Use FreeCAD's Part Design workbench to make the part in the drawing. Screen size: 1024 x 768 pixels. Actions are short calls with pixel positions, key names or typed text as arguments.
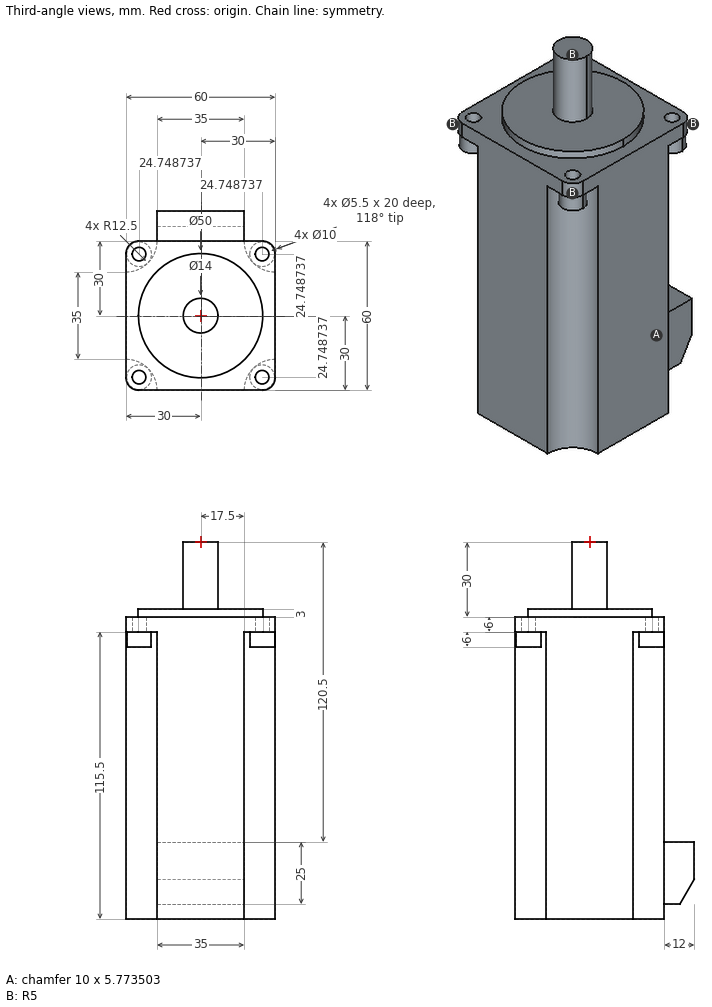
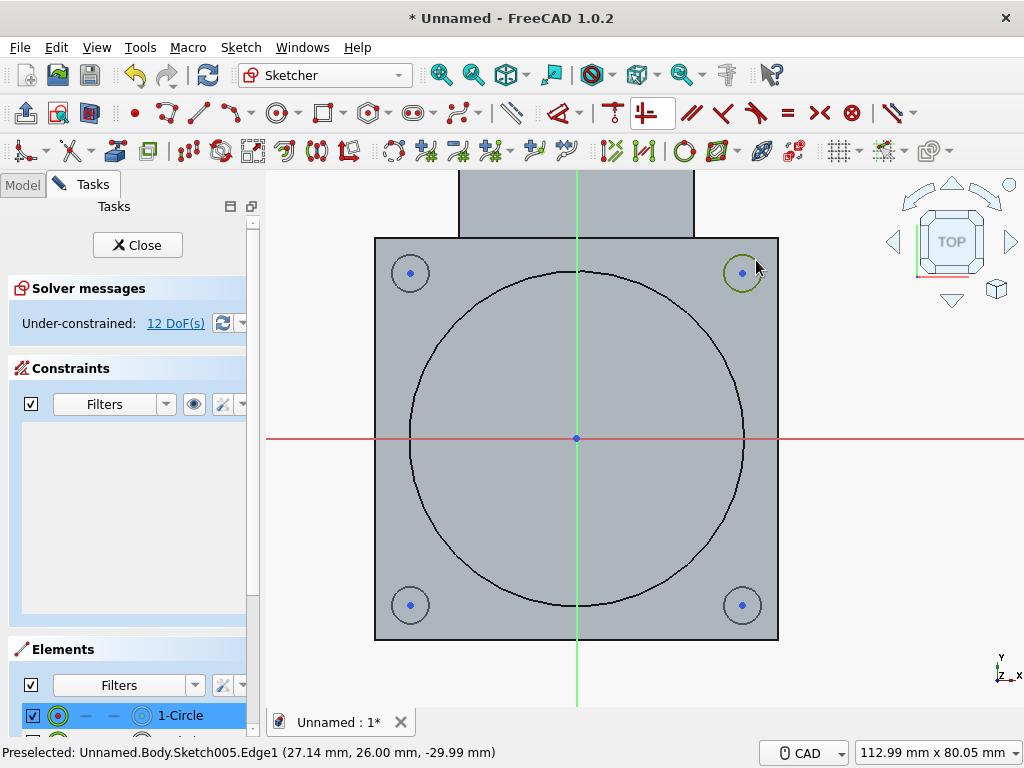
click(423, 260)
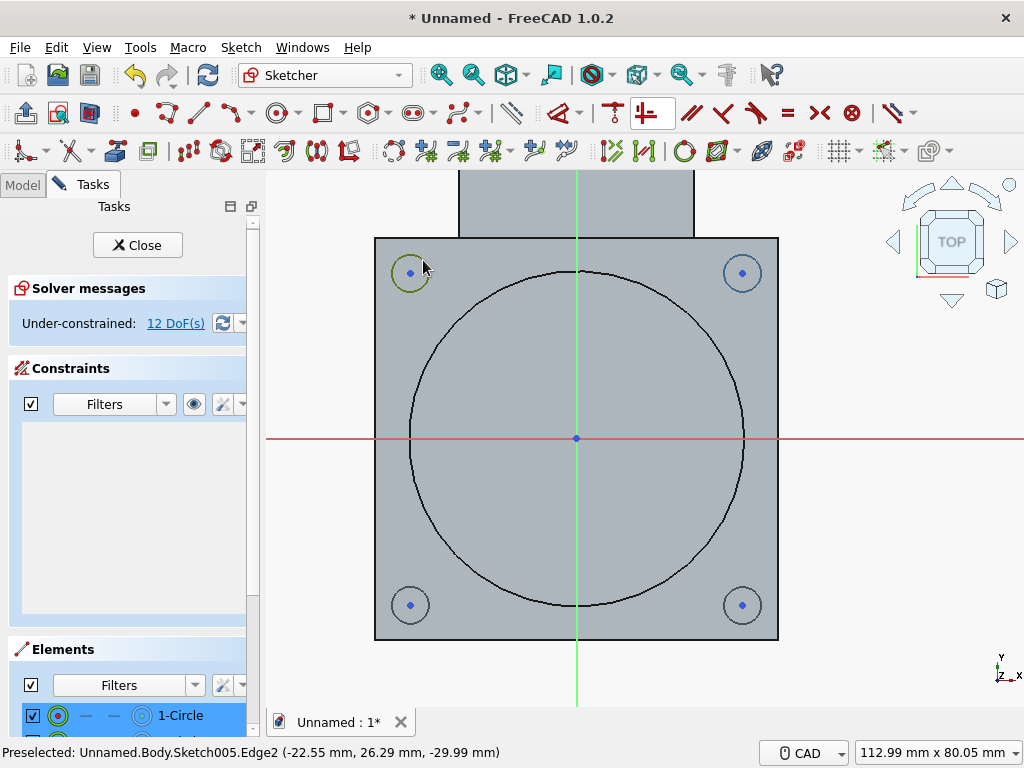
click(756, 592)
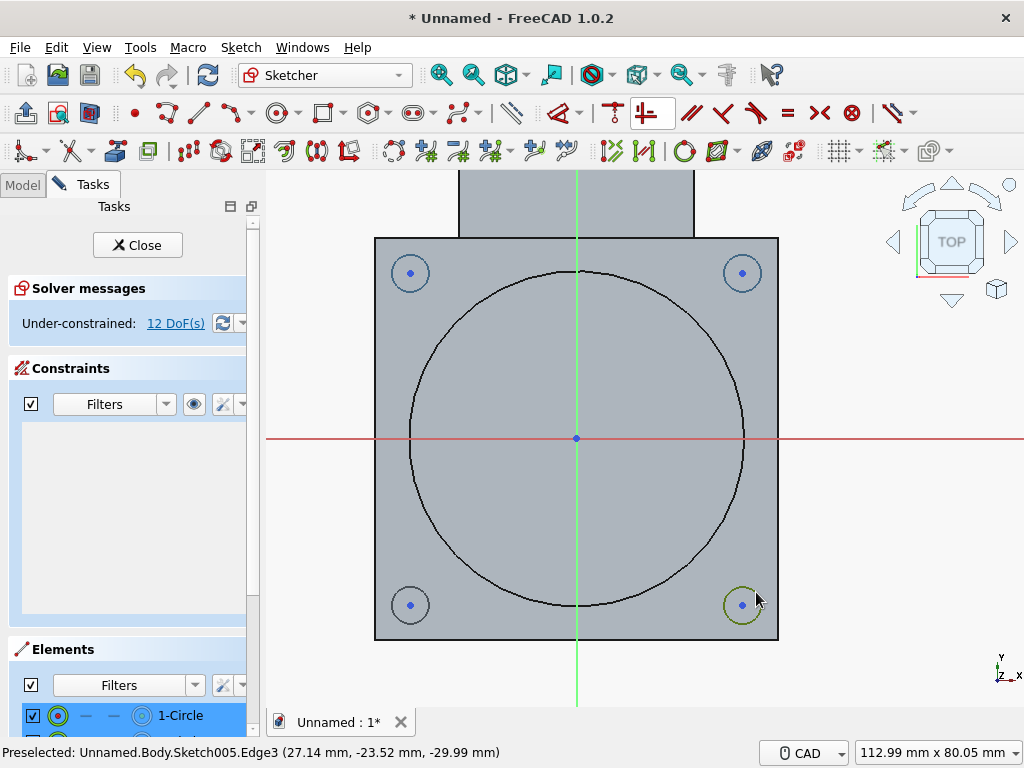
click(423, 592)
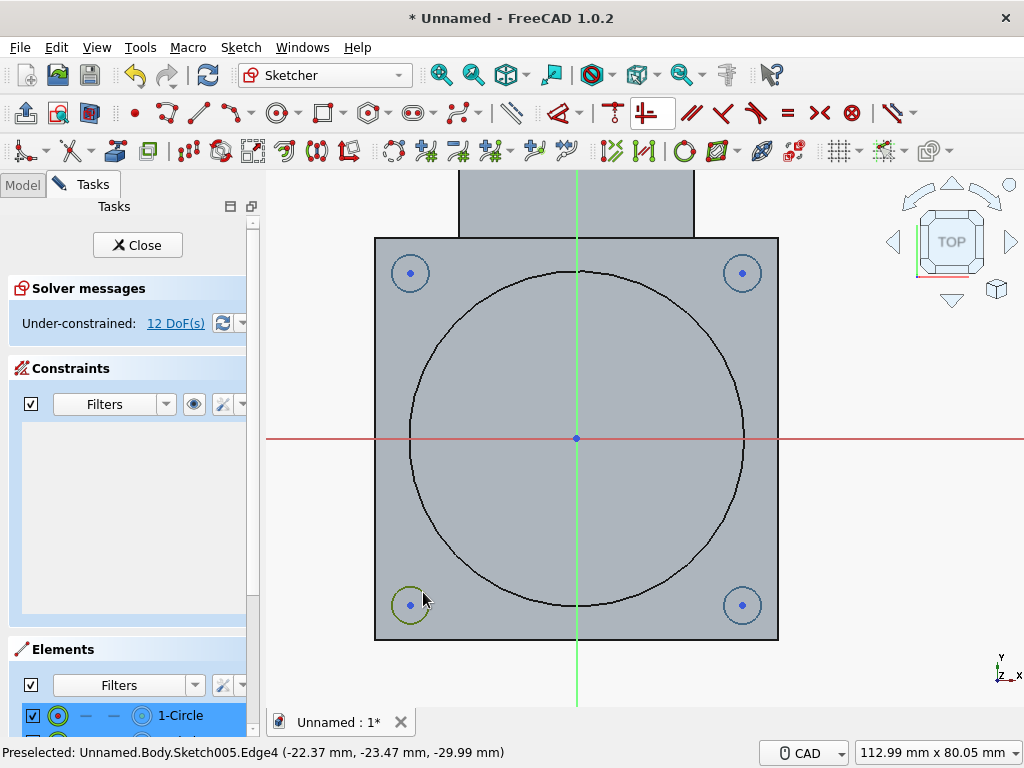
click(788, 114)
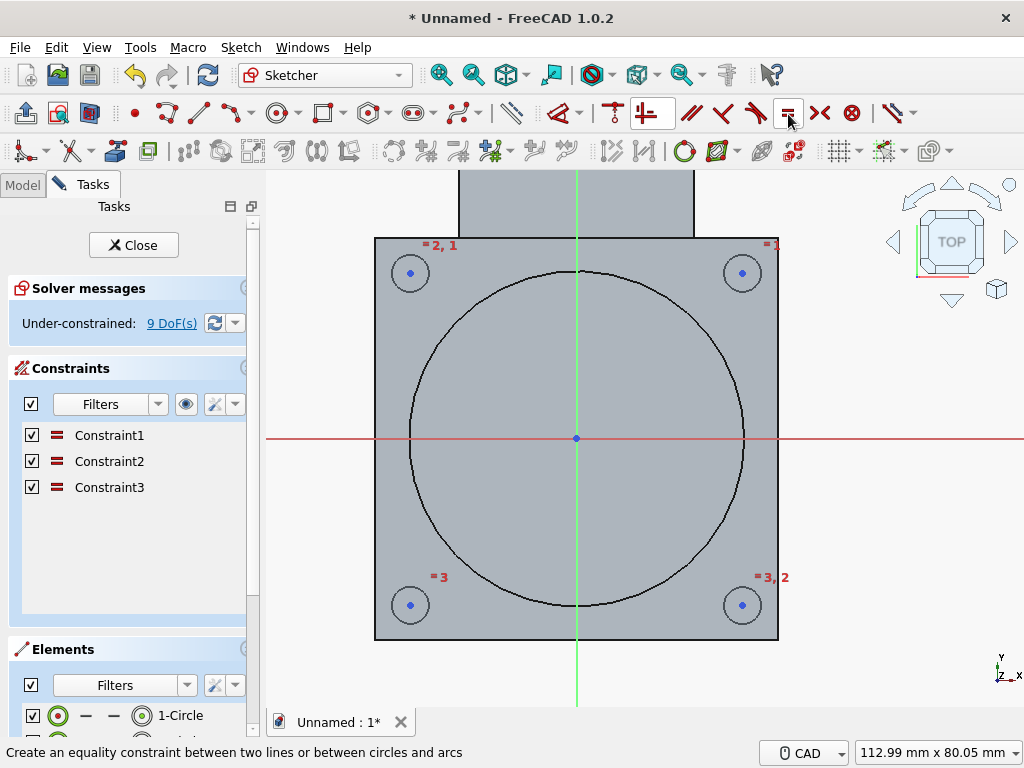
click(743, 273)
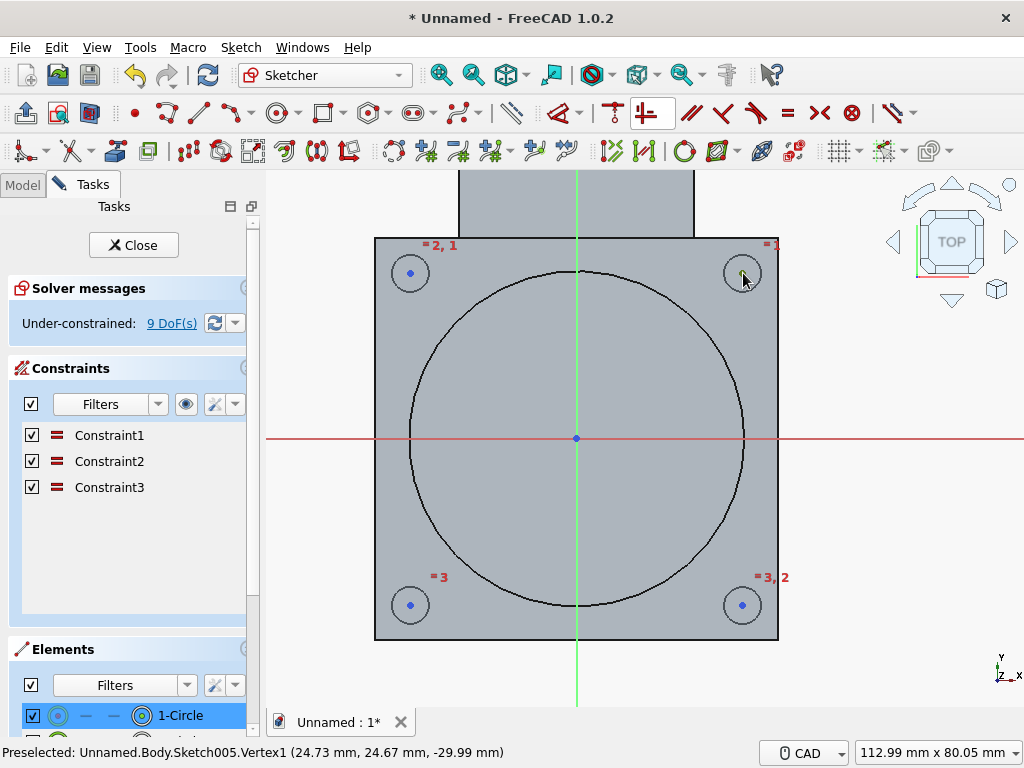
click(410, 273)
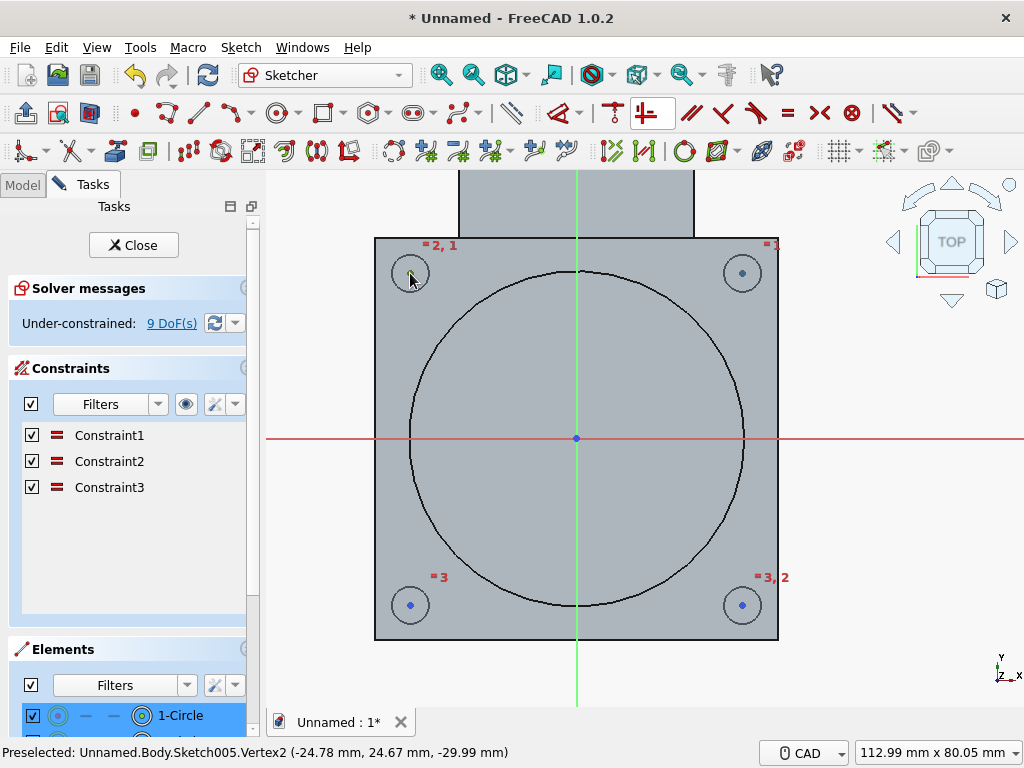
click(670, 114)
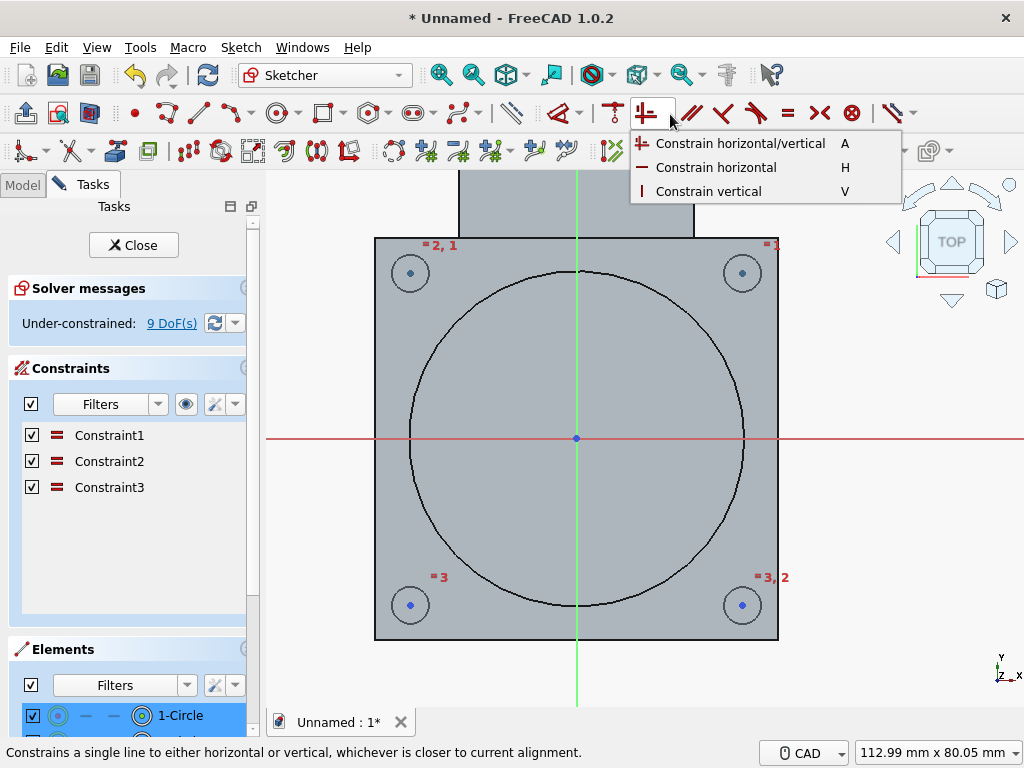
click(766, 167)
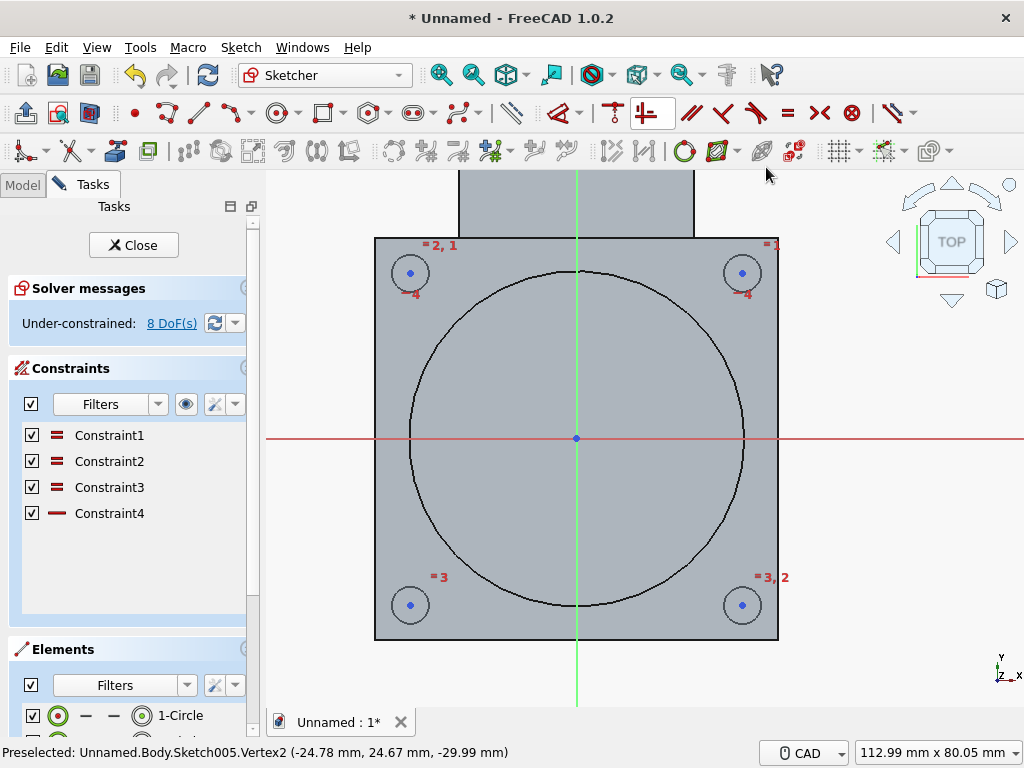
click(743, 273)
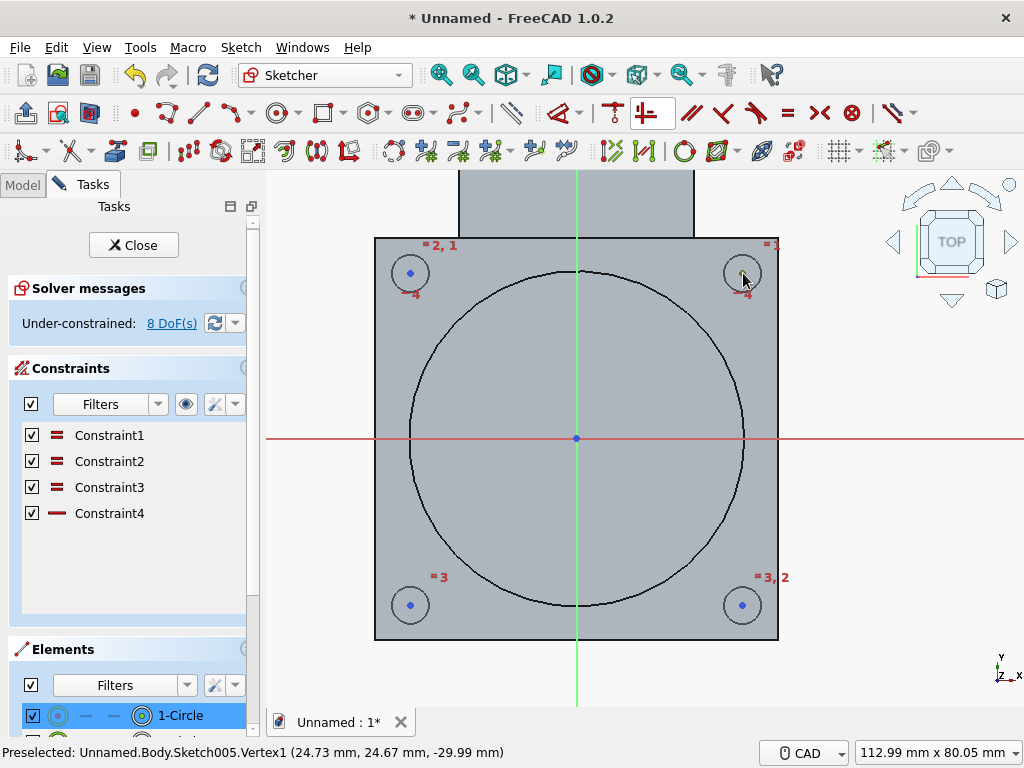
click(743, 606)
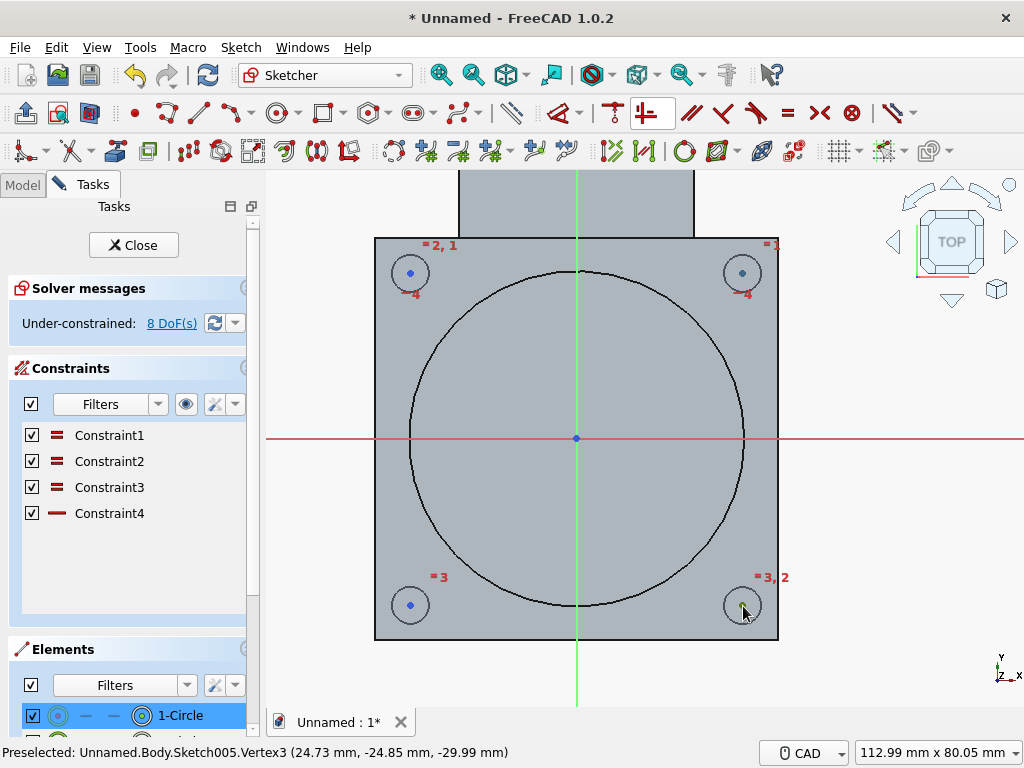
key(v)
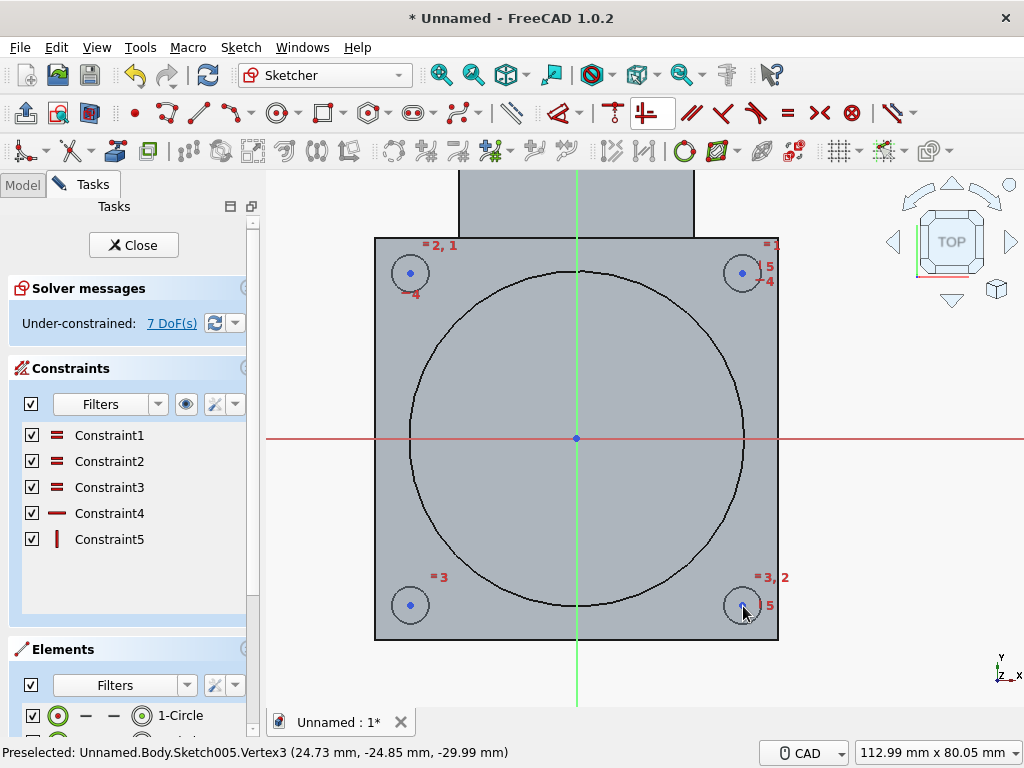
click(410, 273)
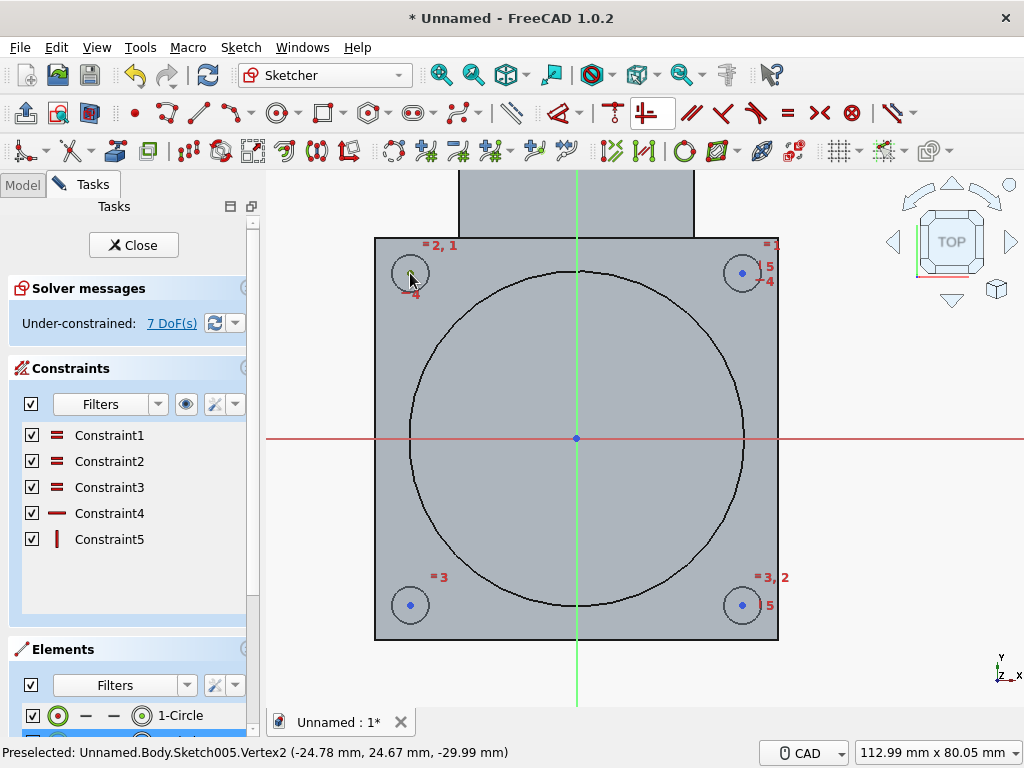
click(410, 605)